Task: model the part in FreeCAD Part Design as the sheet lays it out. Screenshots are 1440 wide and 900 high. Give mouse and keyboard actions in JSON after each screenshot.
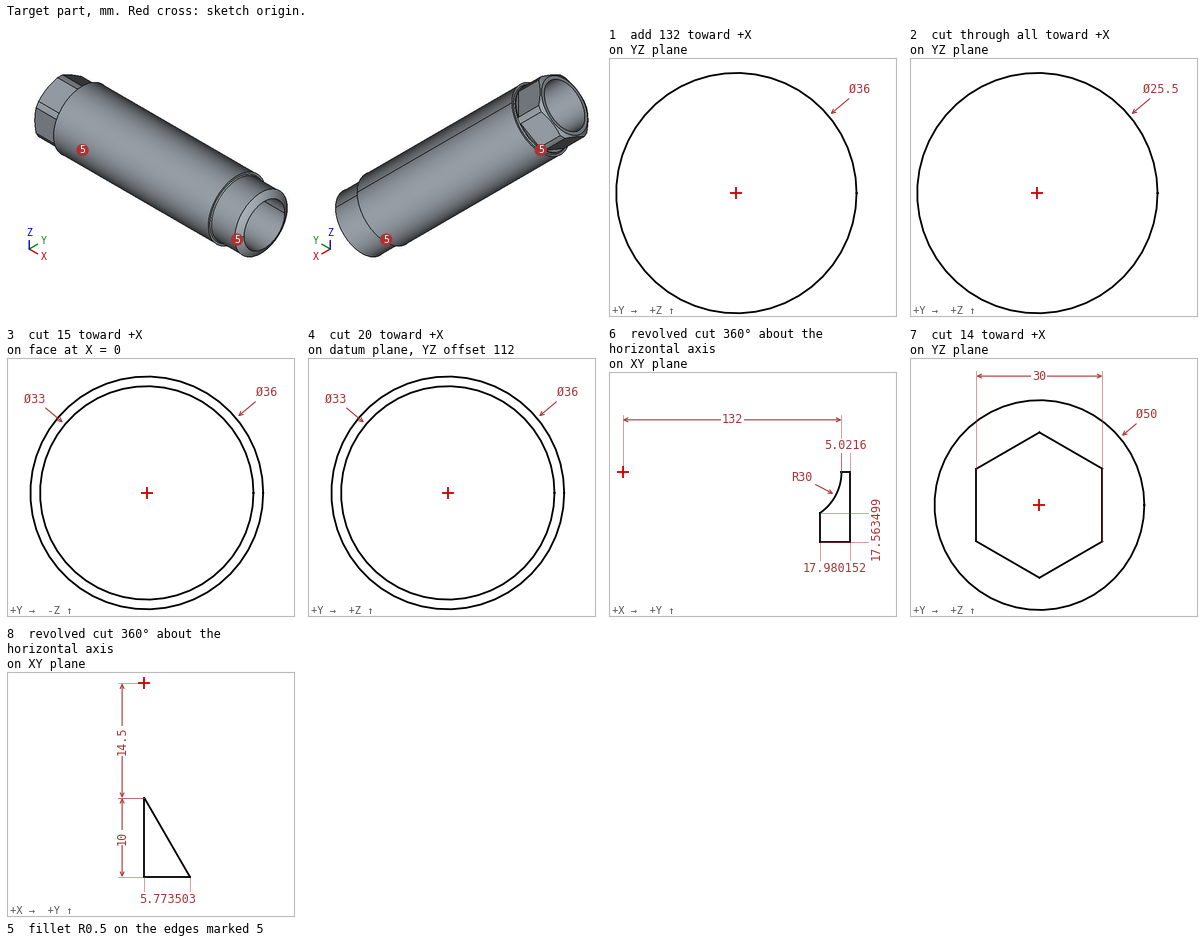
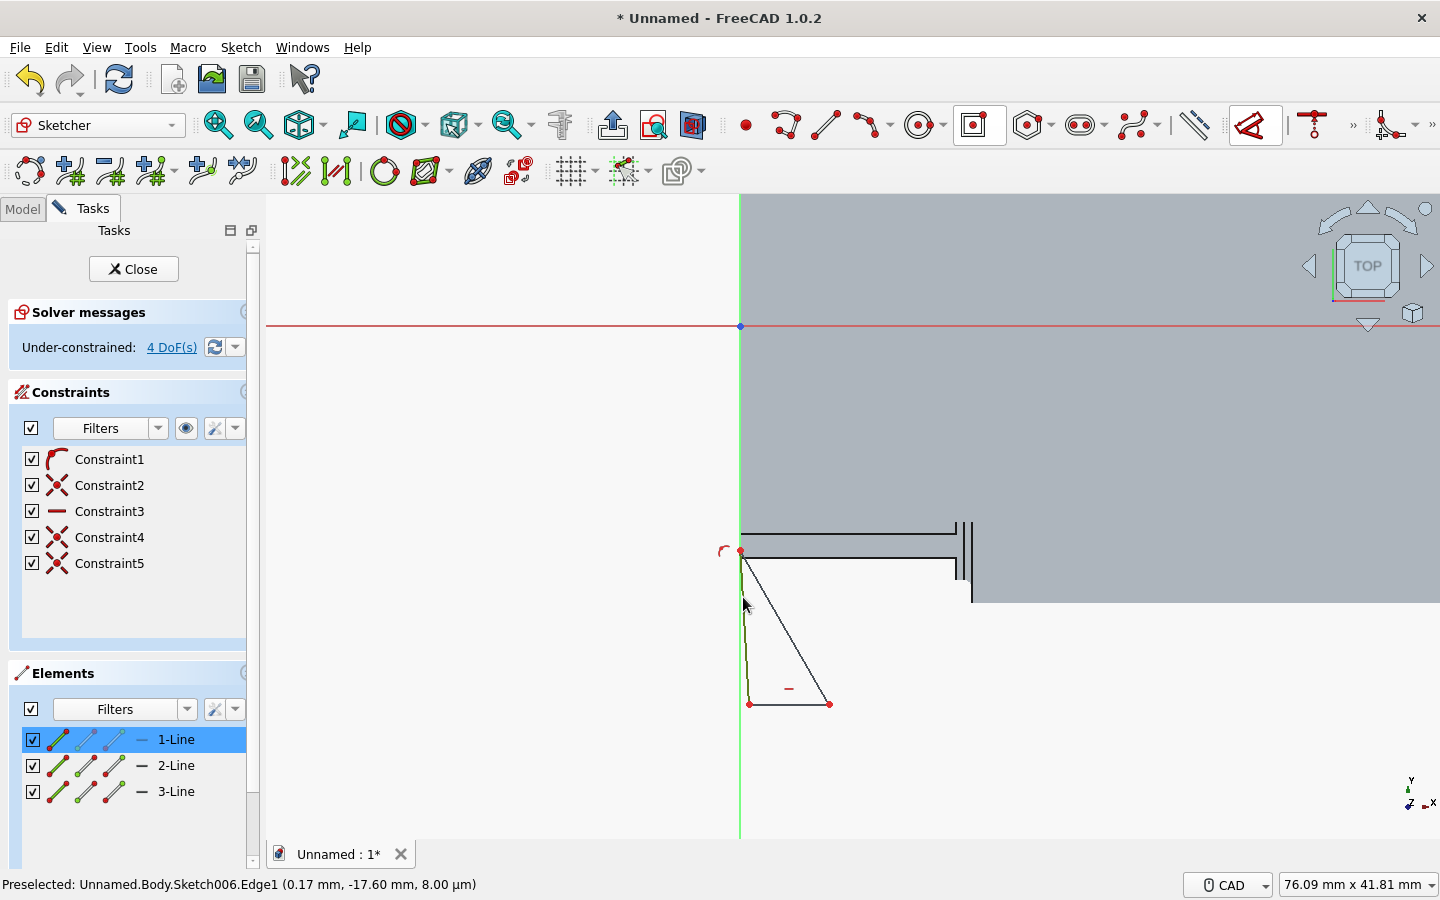
{"action": "key", "text": "v"}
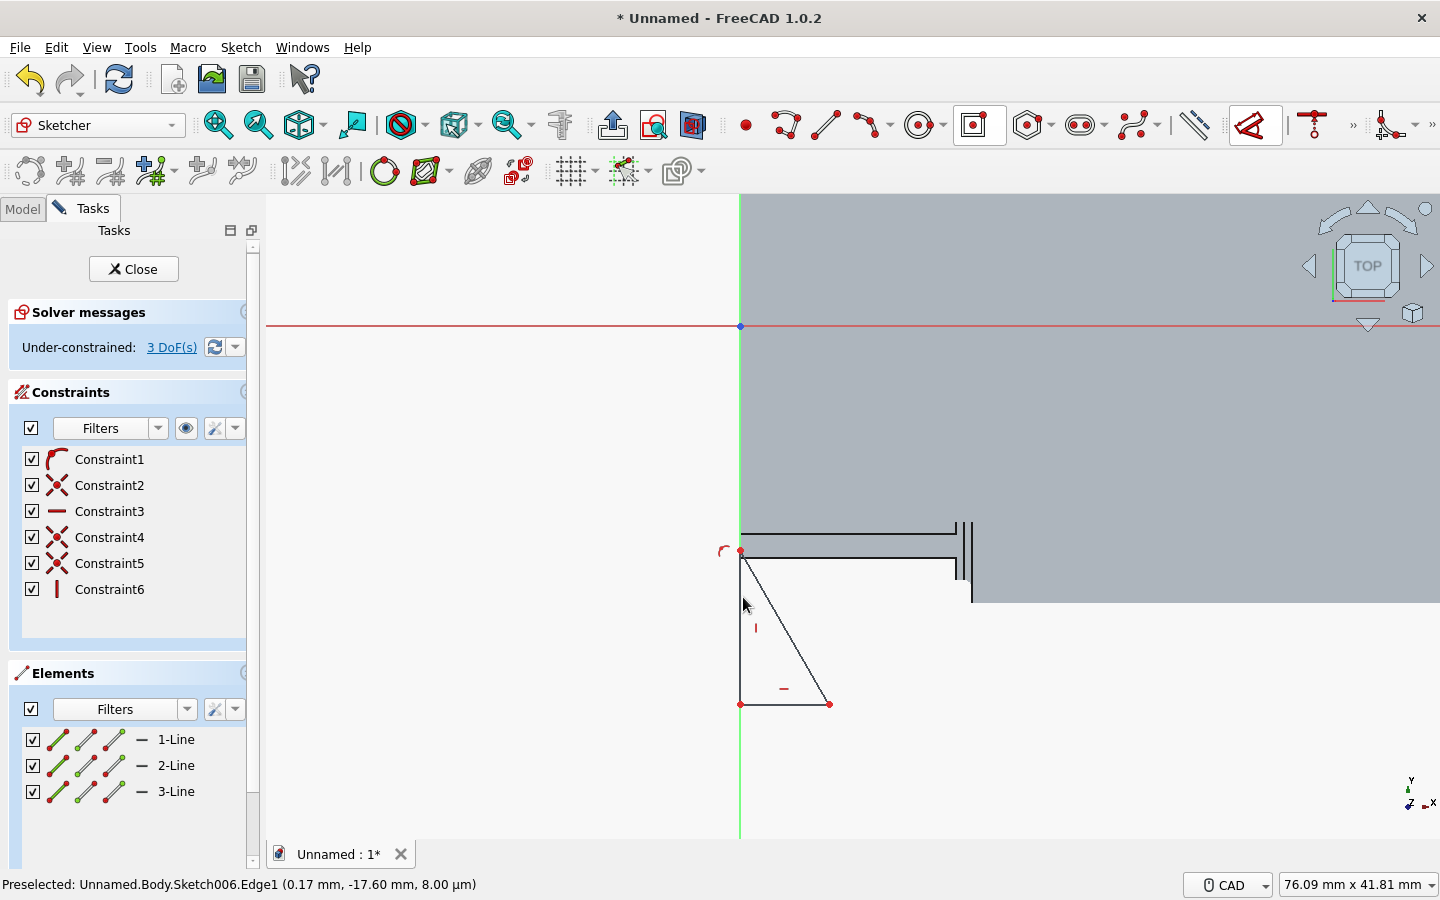
{"action": "left_click", "coordinate": [740, 597]}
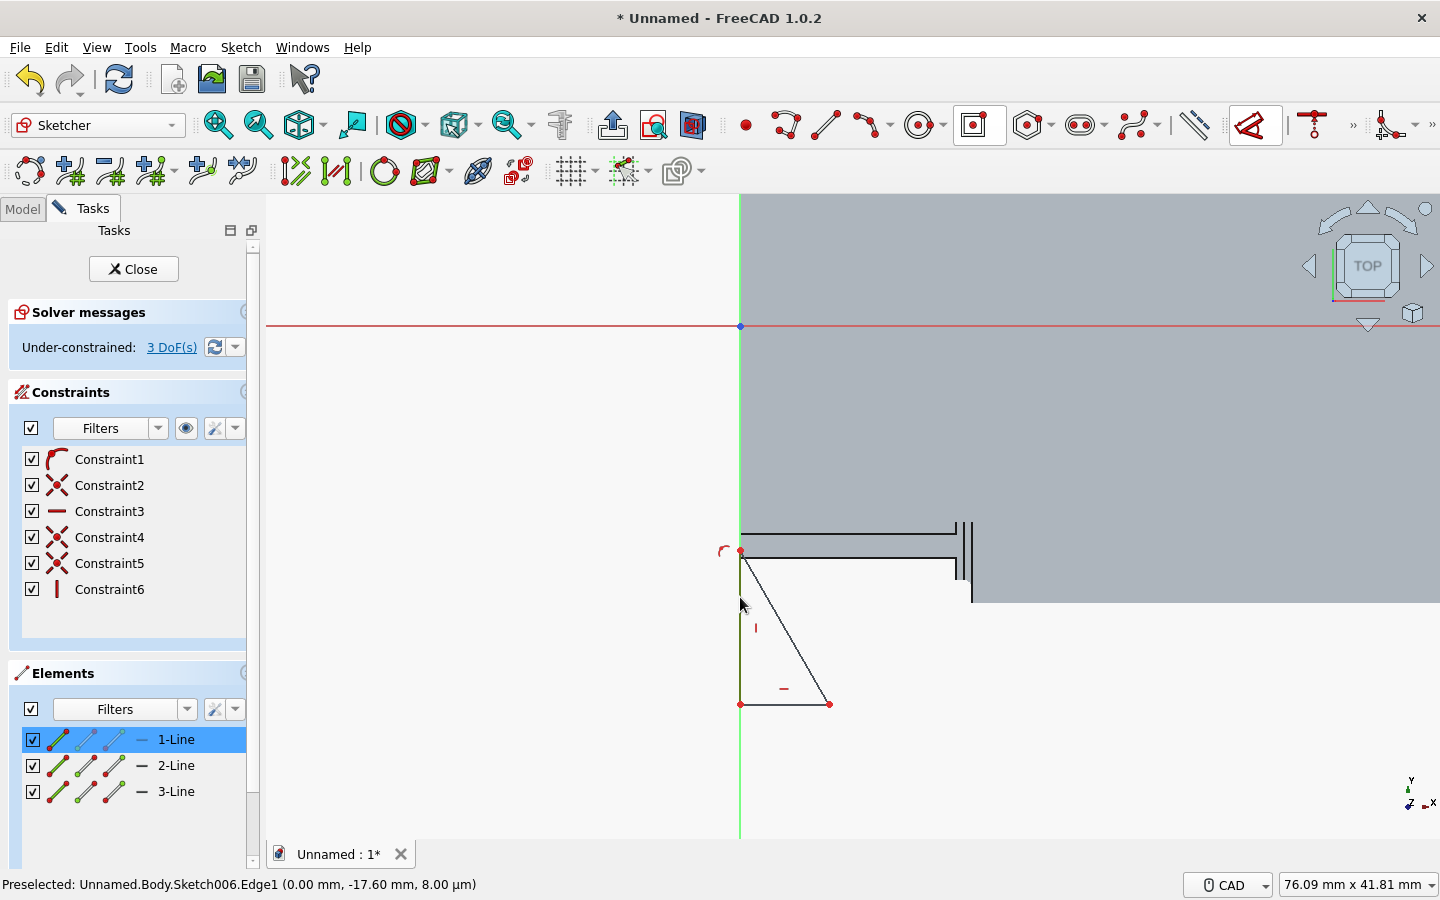
{"action": "left_click", "coordinate": [1276, 126]}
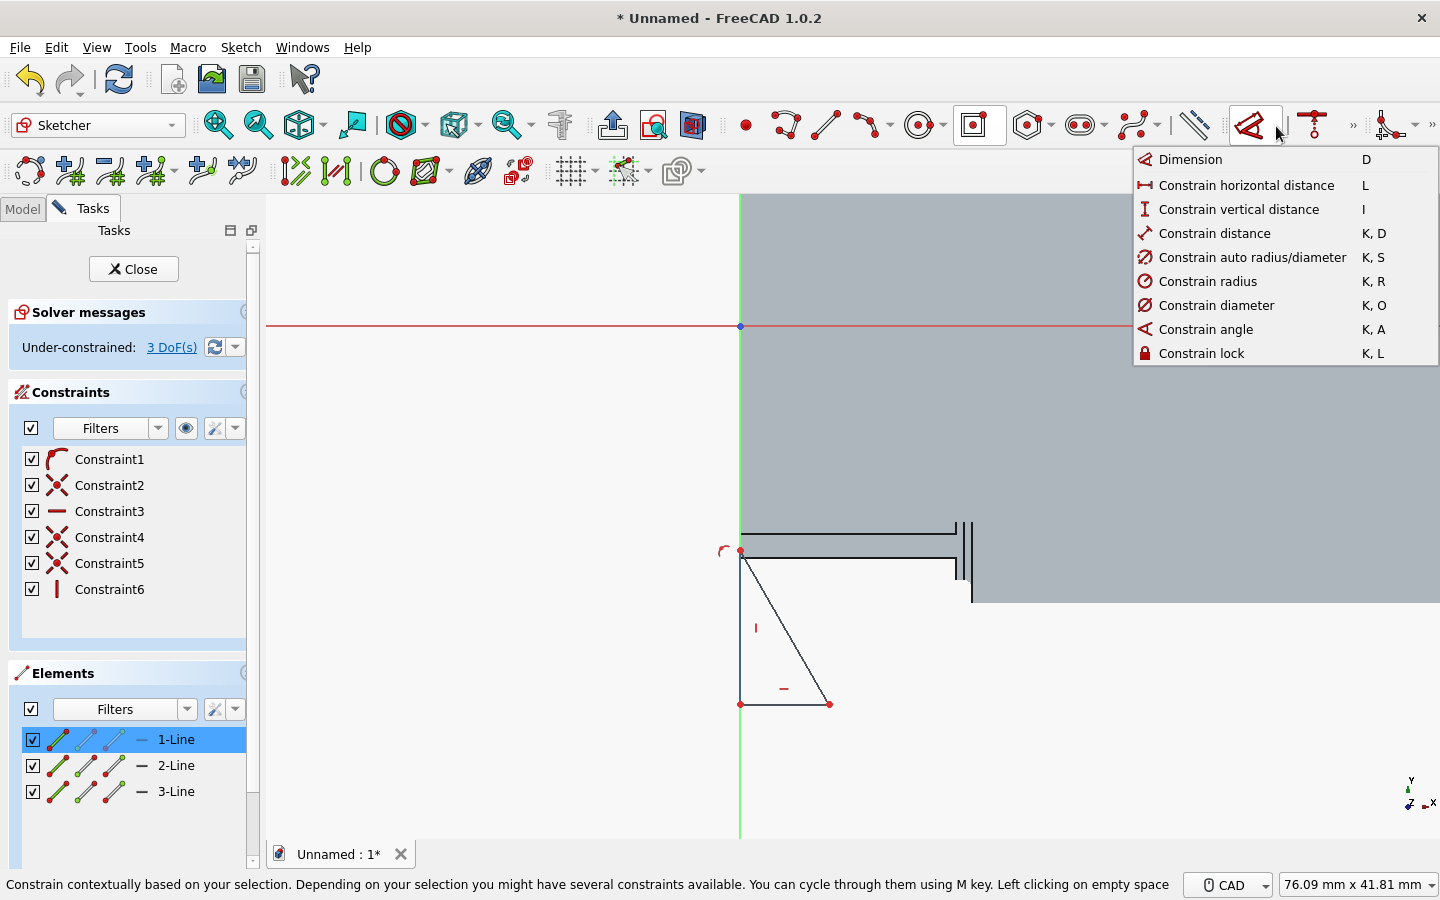
{"action": "left_click", "coordinate": [1286, 209]}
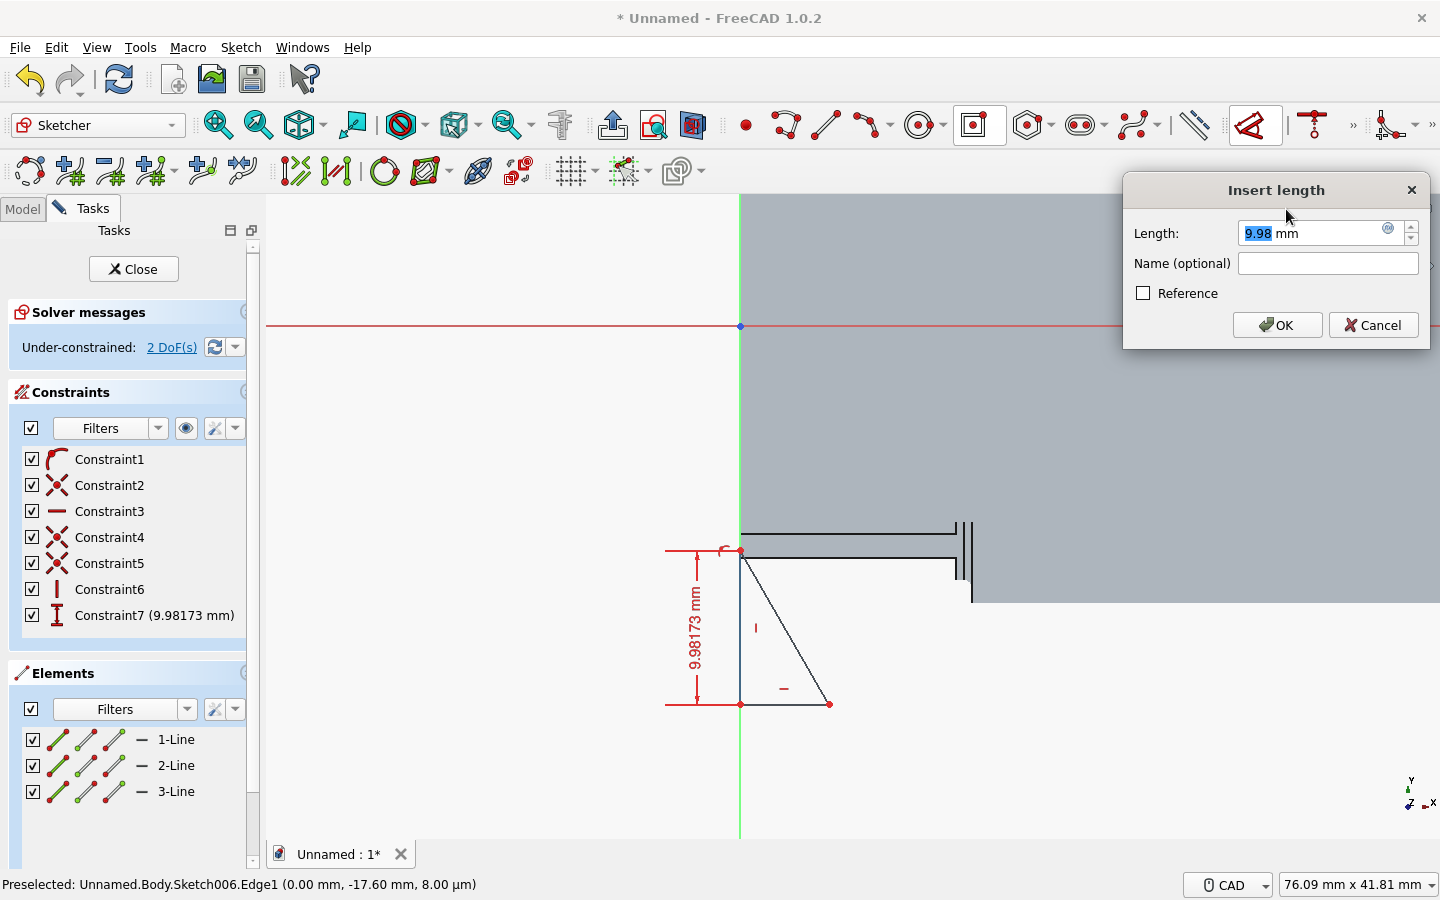
{"action": "type", "text": "10"}
{"action": "key", "text": "Return"}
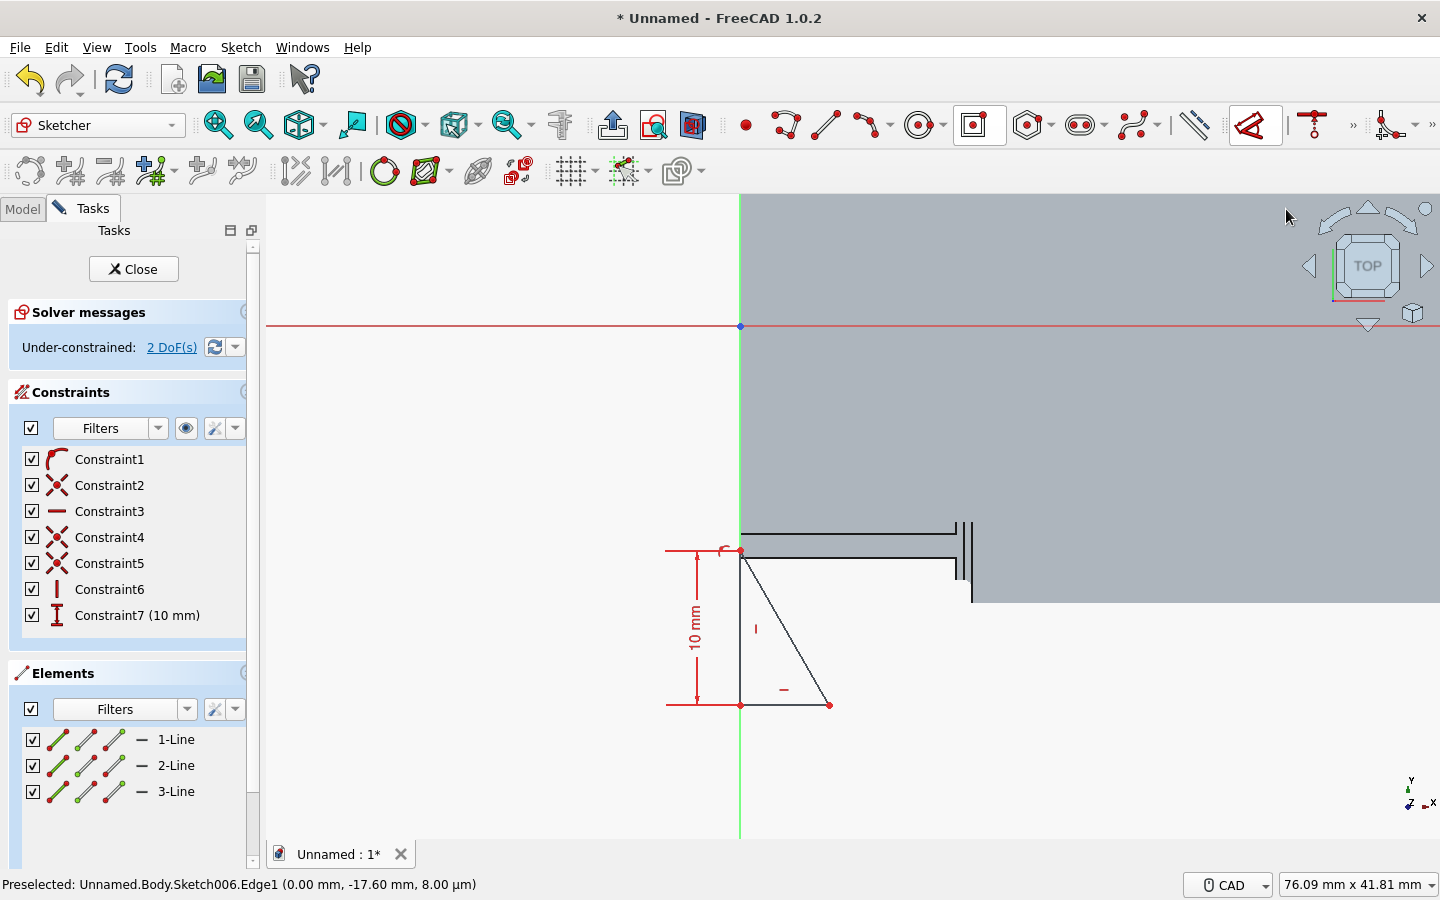
{"action": "left_click", "coordinate": [740, 551]}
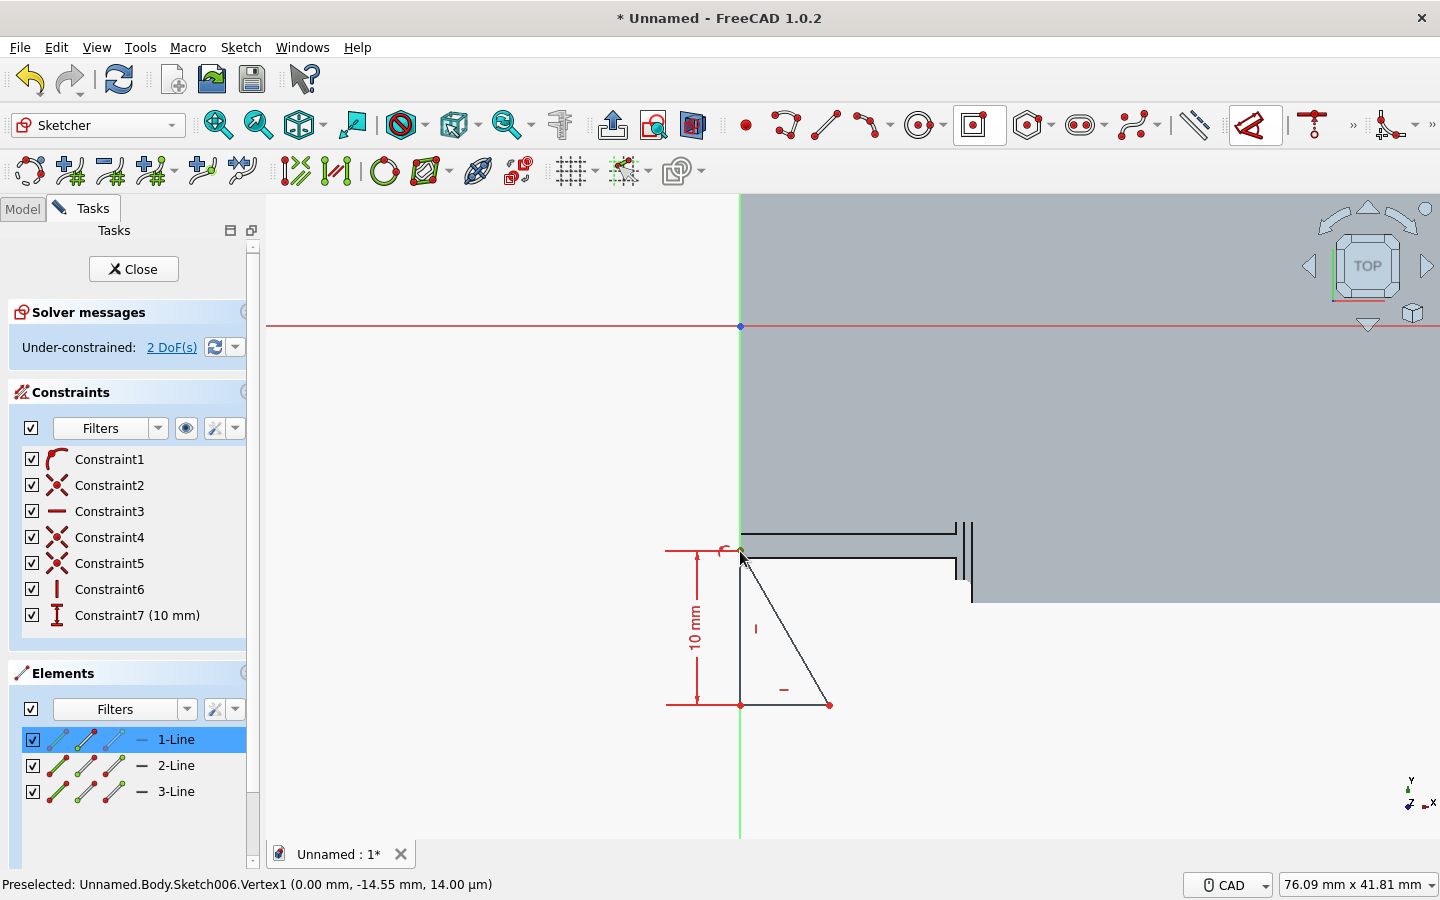
{"action": "left_click", "coordinate": [1276, 126]}